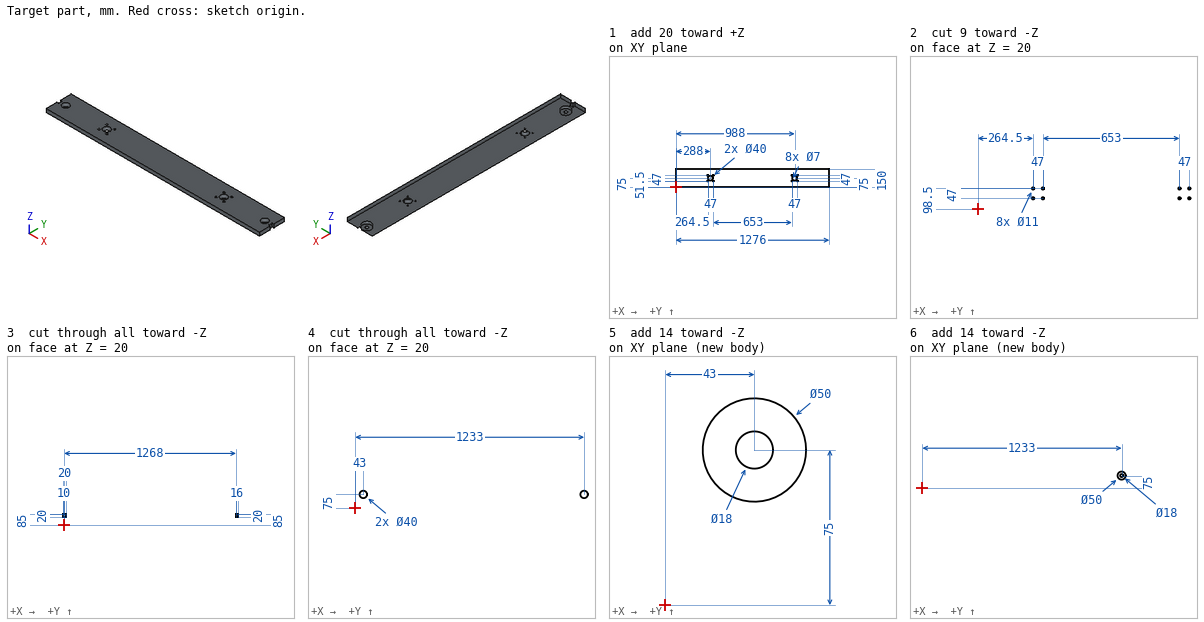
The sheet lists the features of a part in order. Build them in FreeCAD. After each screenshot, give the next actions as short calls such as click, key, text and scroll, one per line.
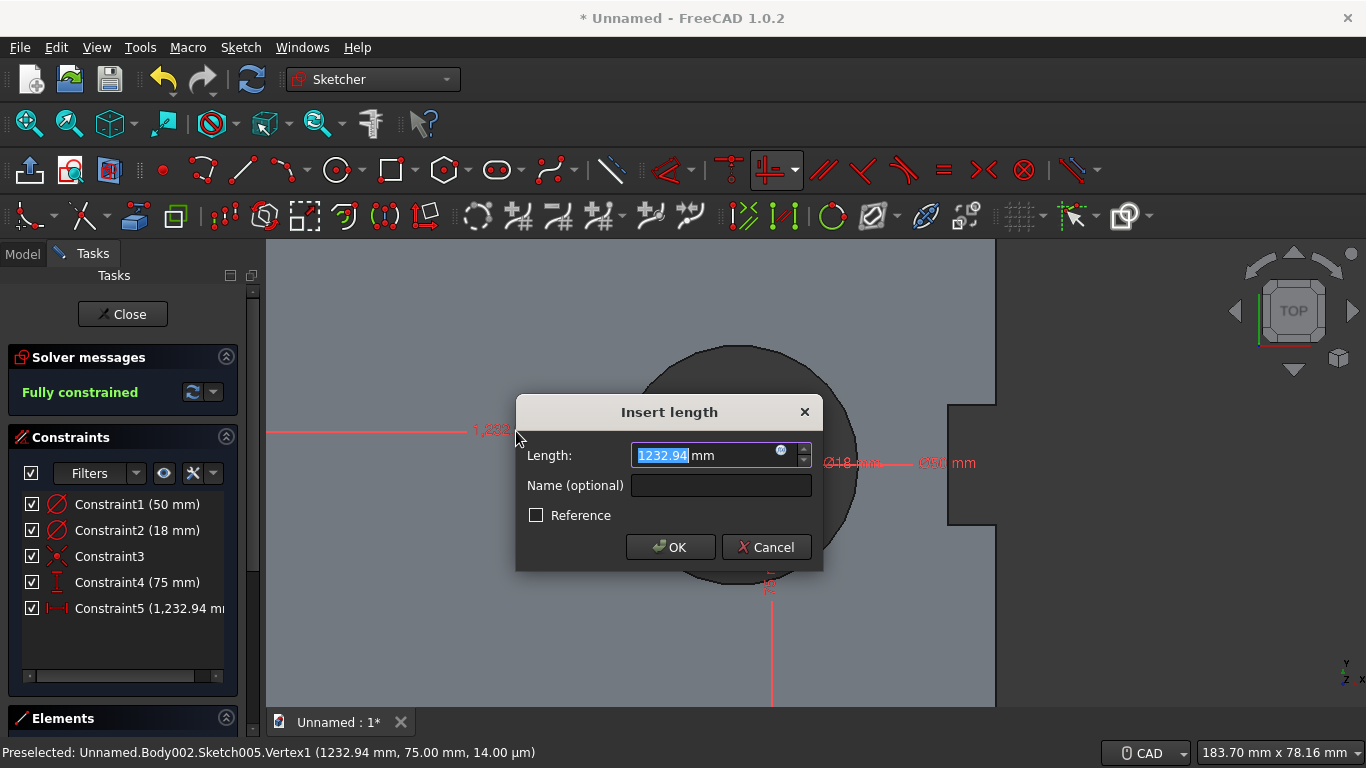
text(1233)
key(Return)
key(Escape)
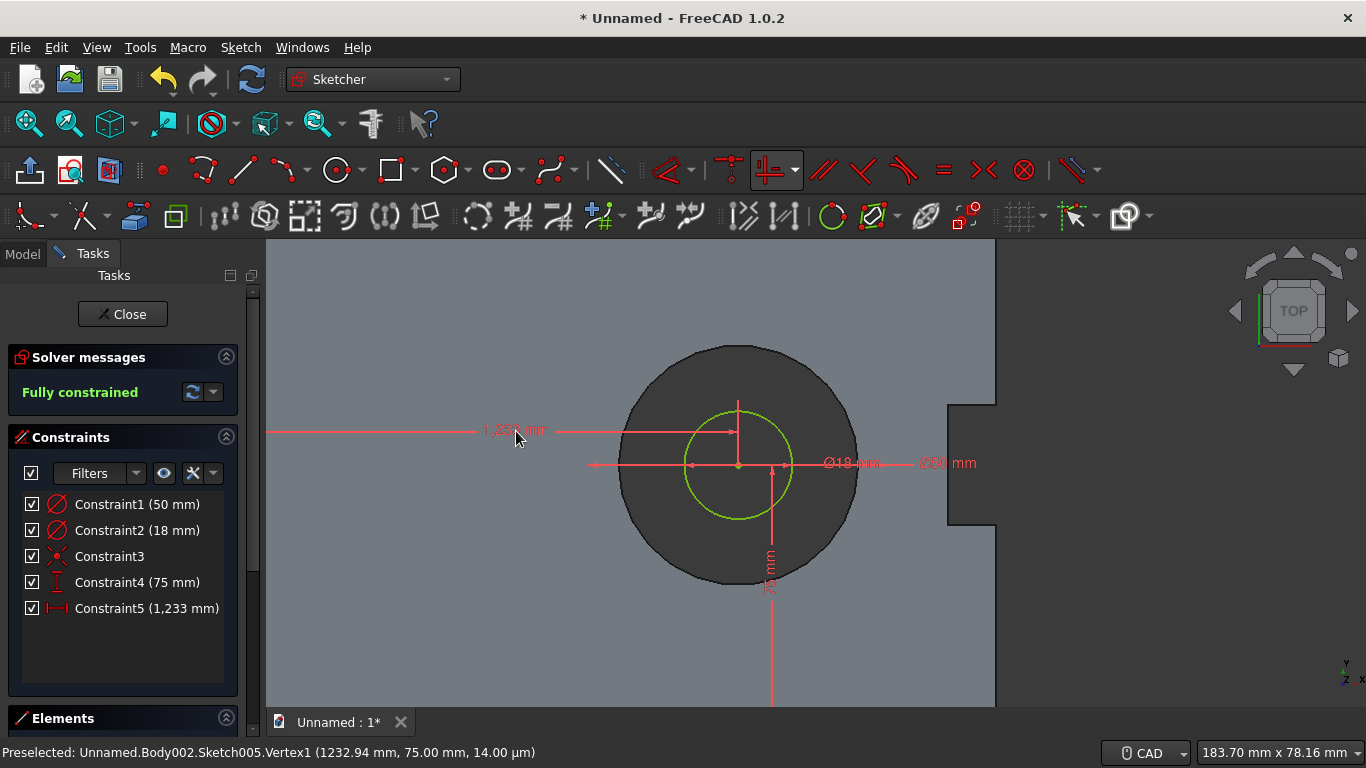
click(123, 314)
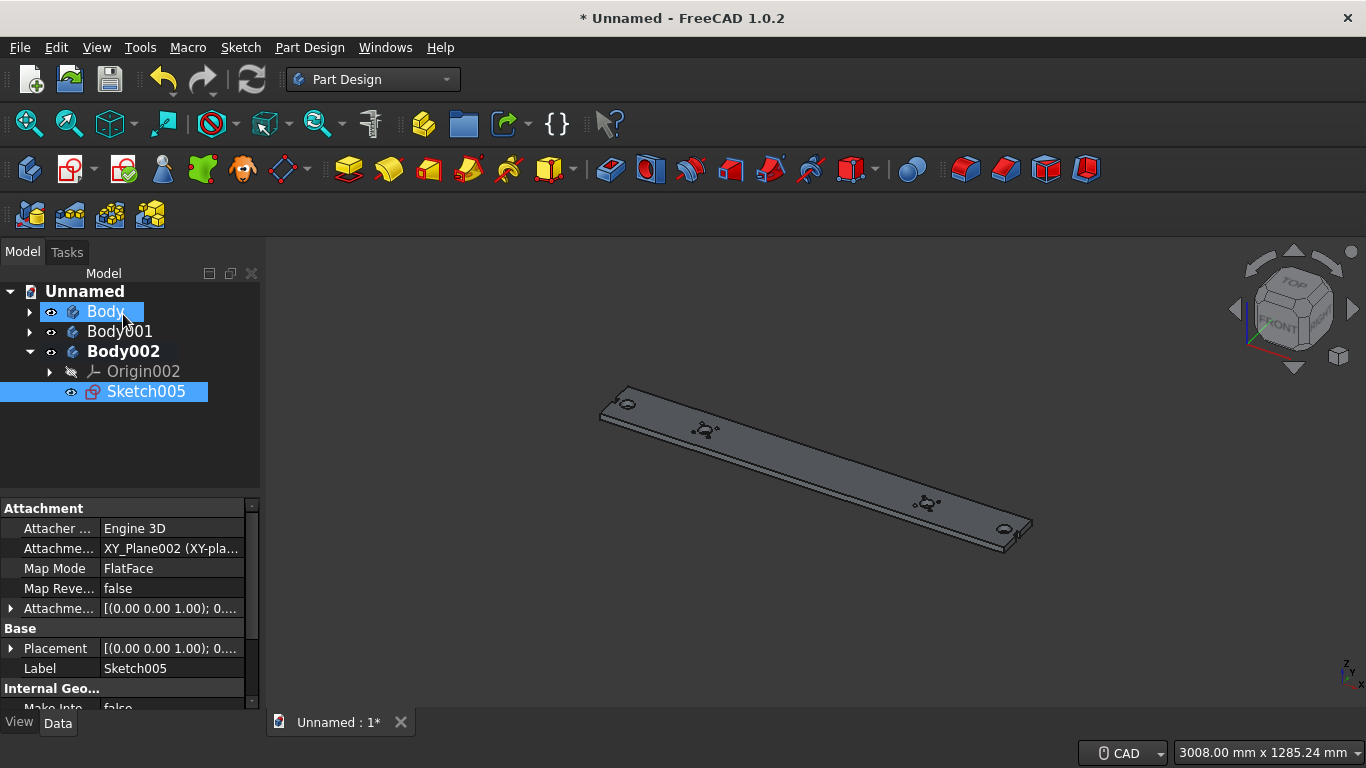
click(350, 170)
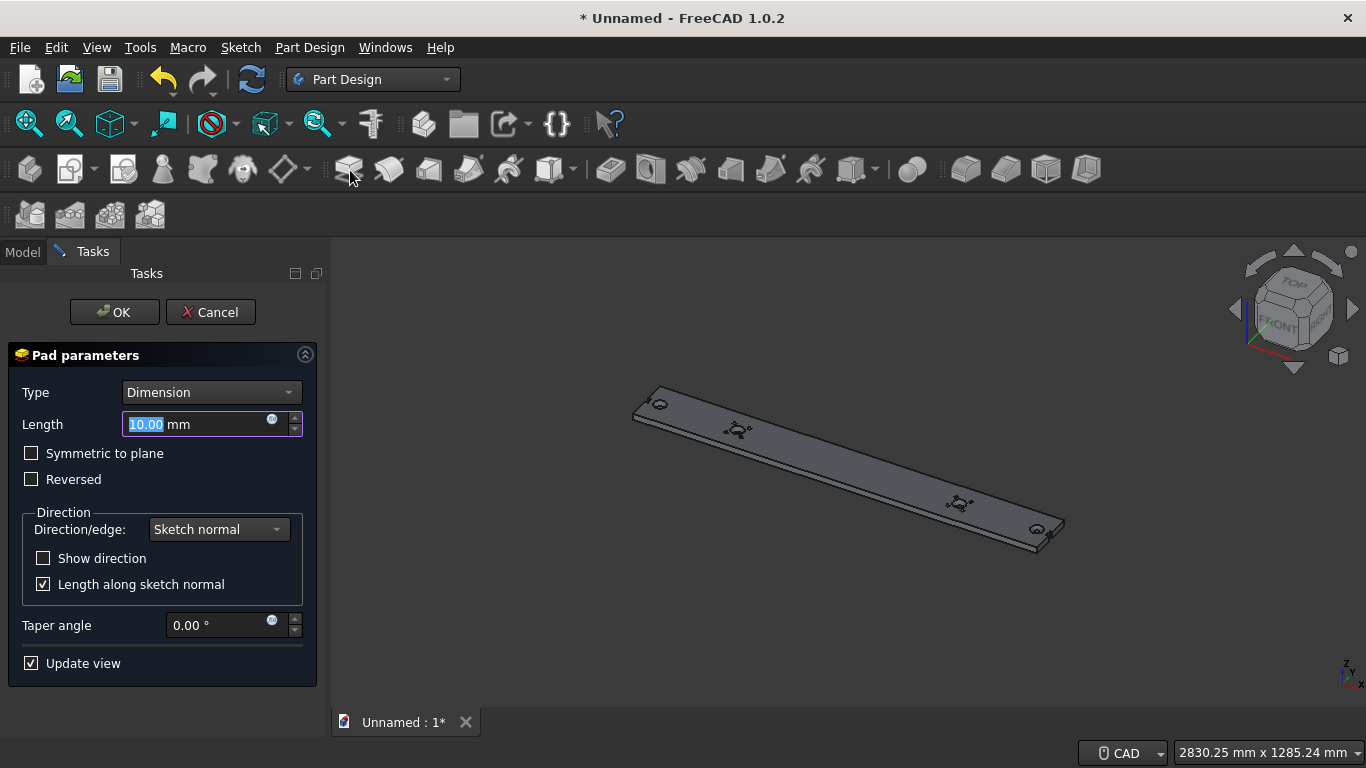
text(14)
key(Tab)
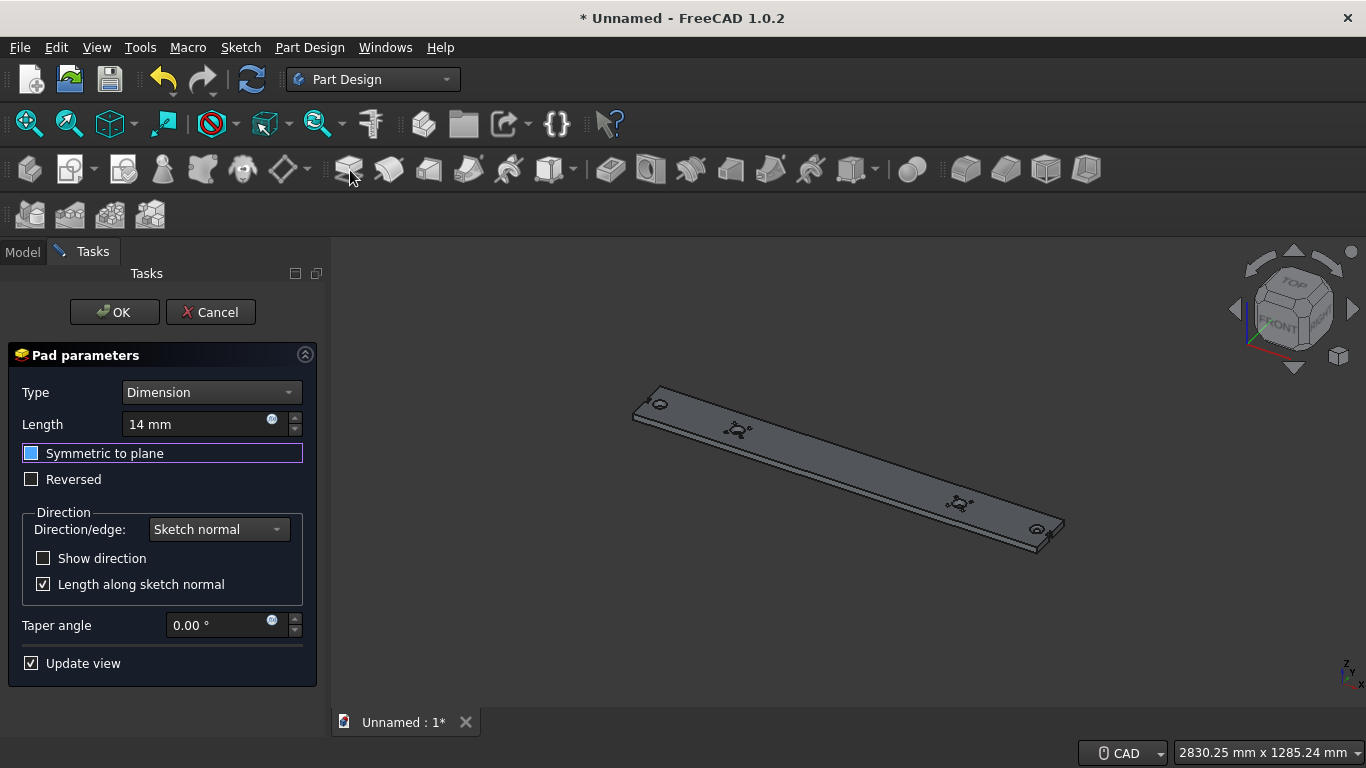
click(30, 479)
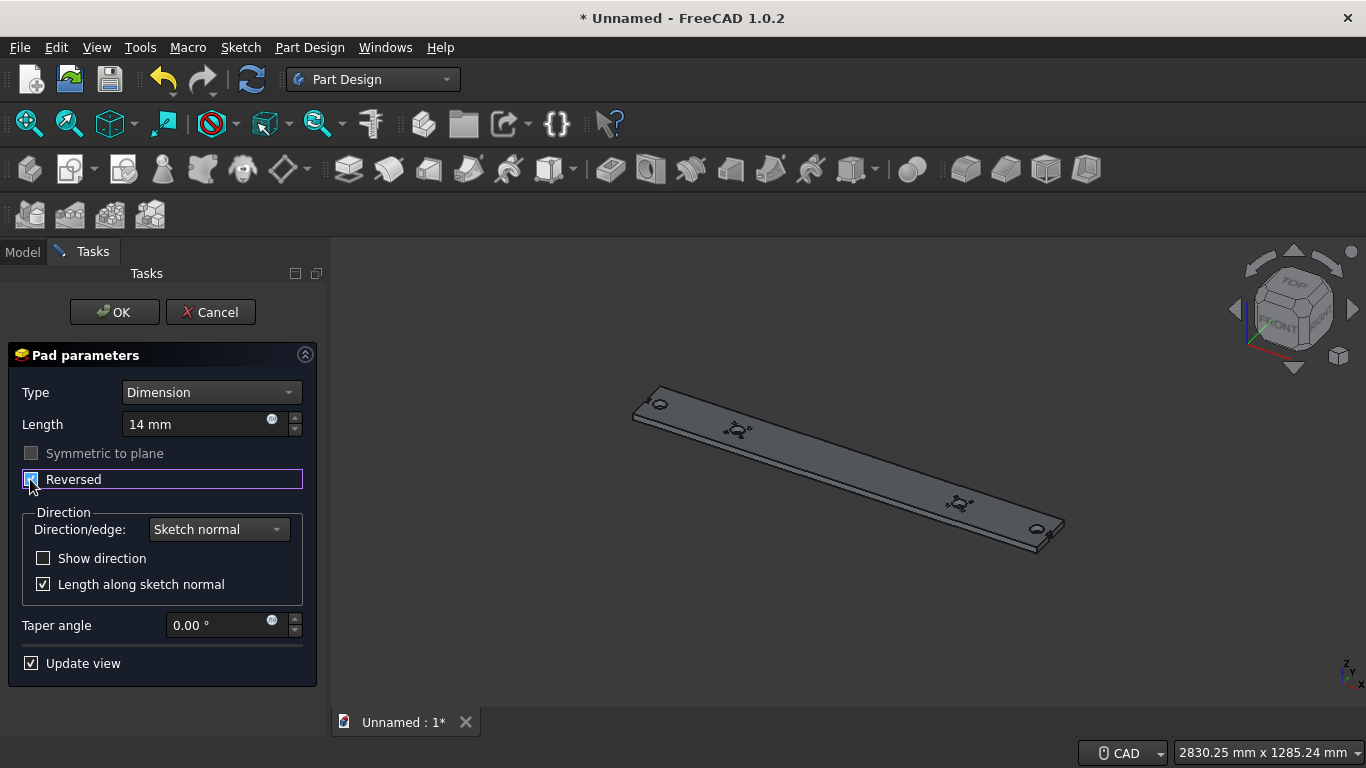
click(115, 312)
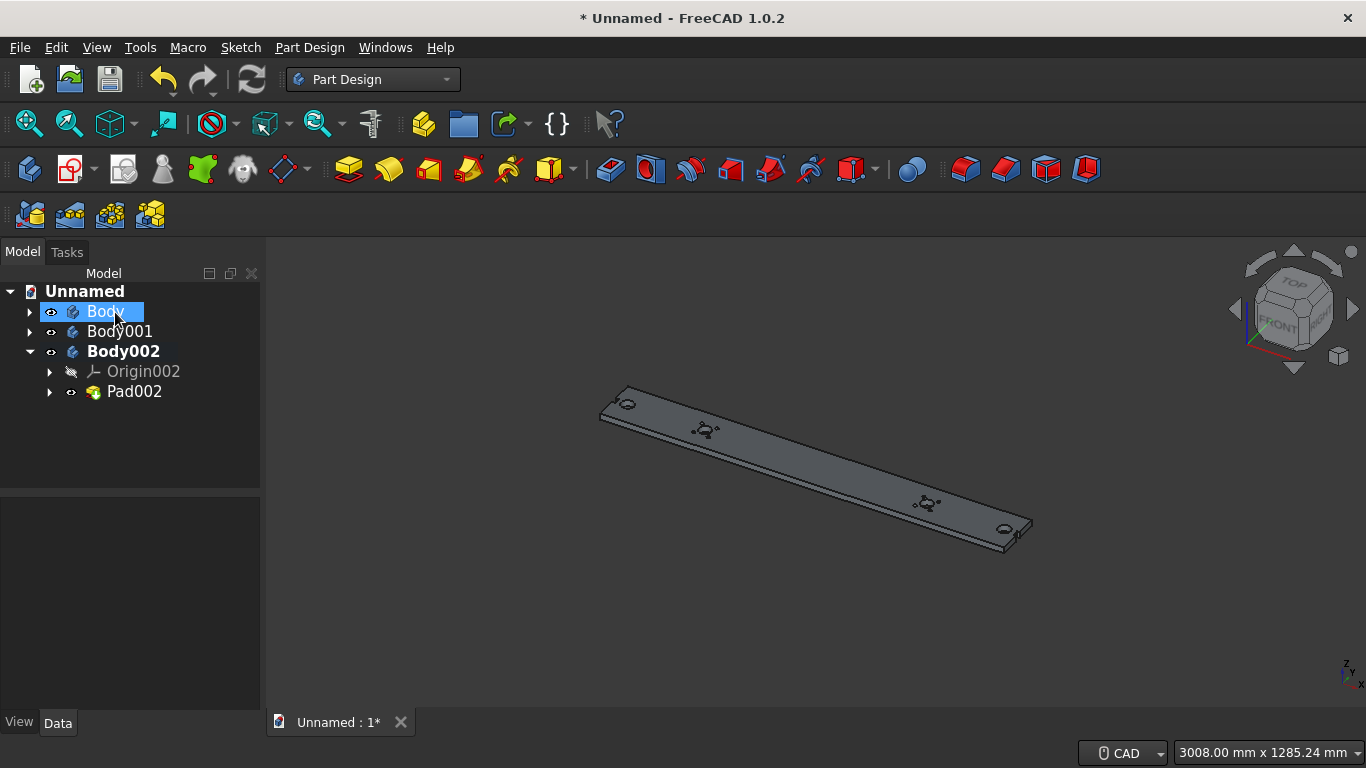
key(0)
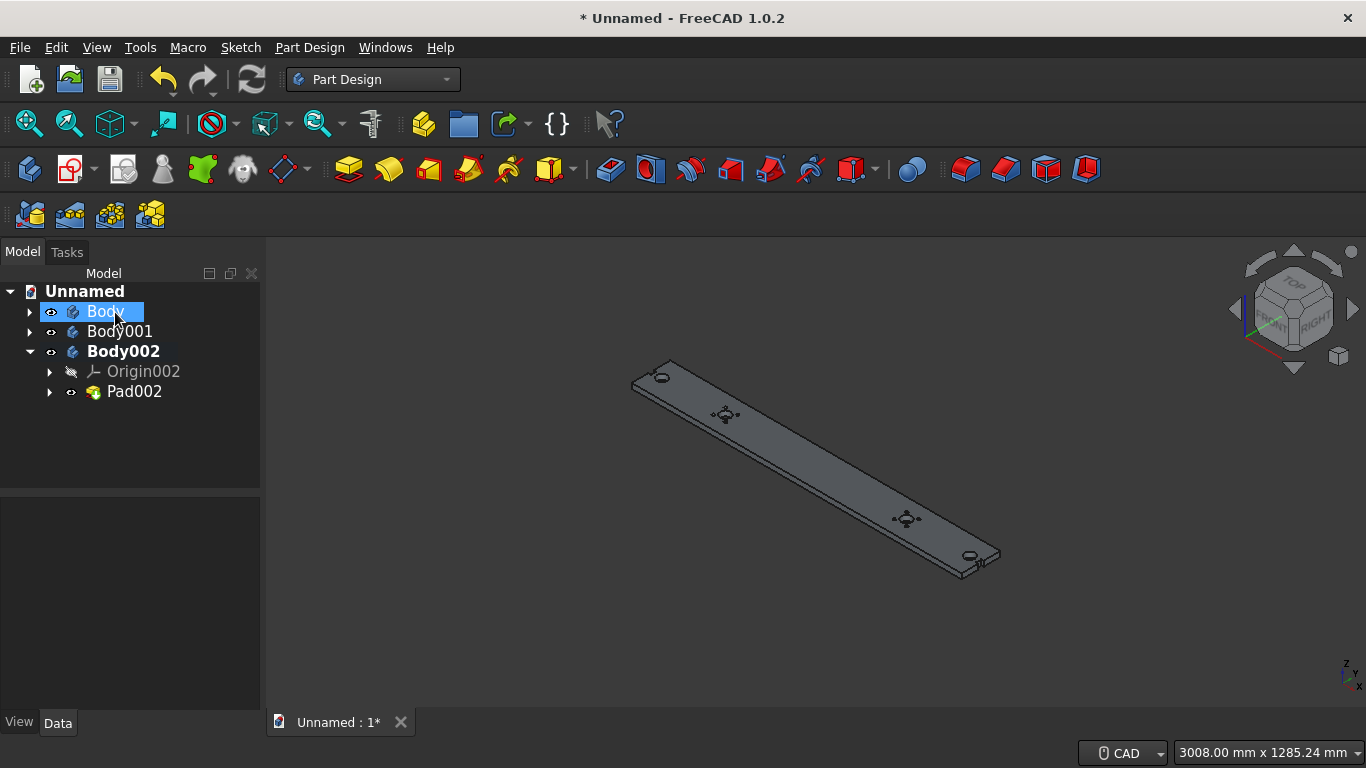
click(30, 124)